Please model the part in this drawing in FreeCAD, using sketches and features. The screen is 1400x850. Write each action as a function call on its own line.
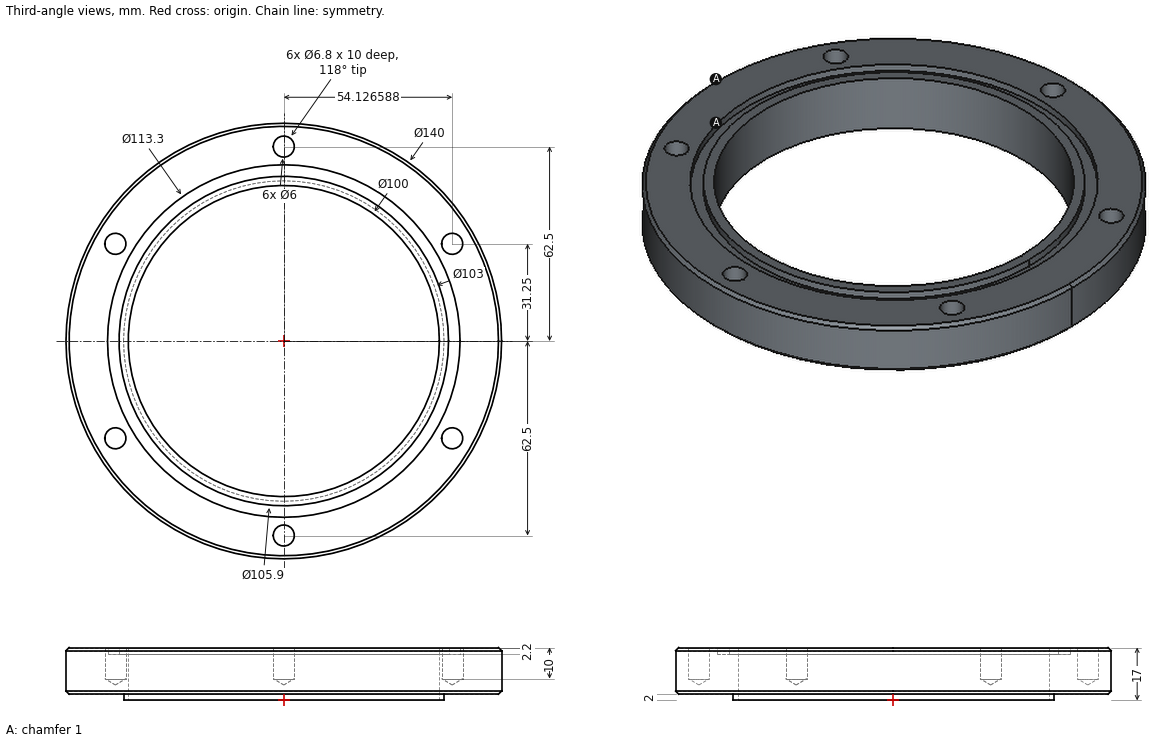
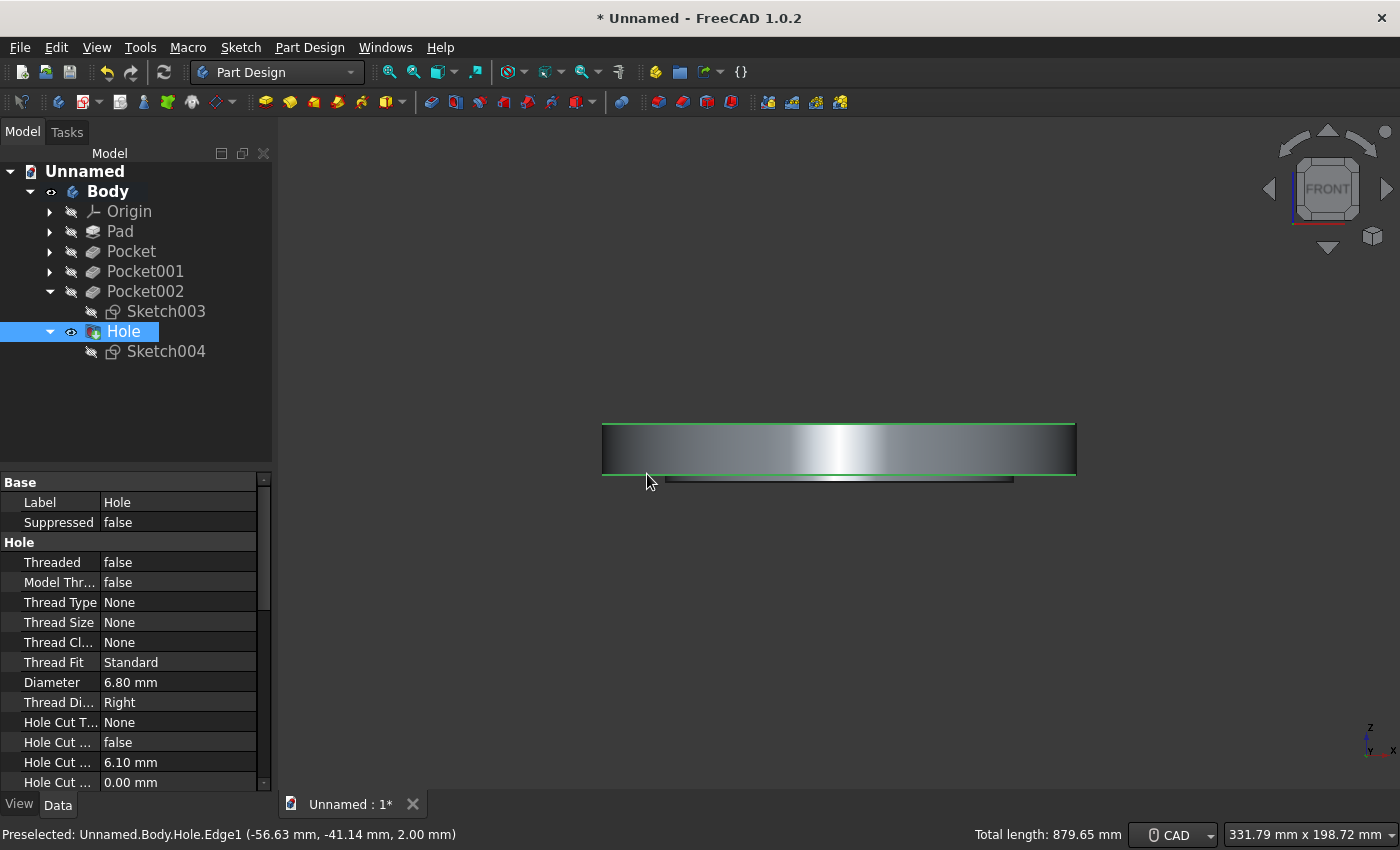
click(684, 102)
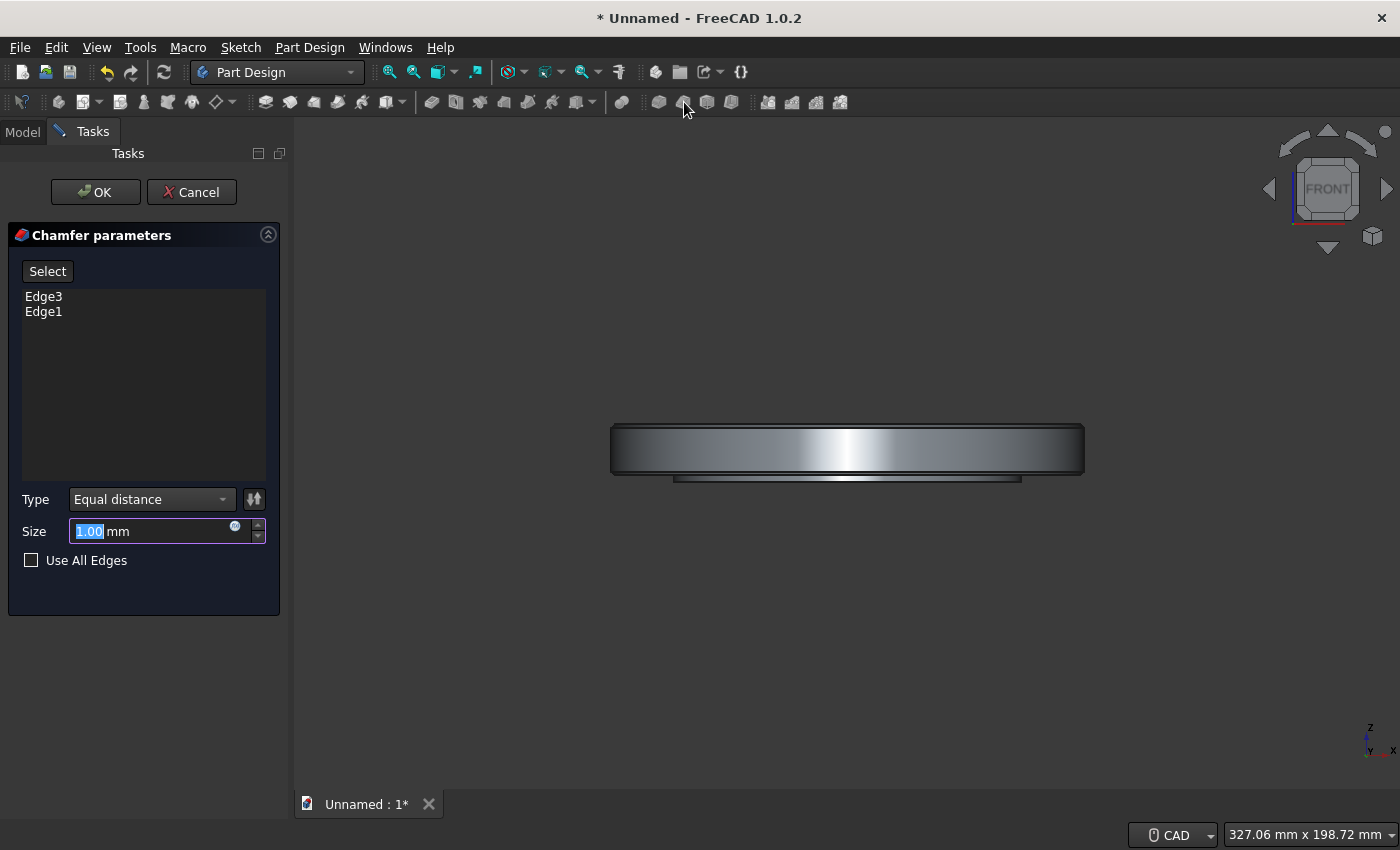
text(1)
key(Tab)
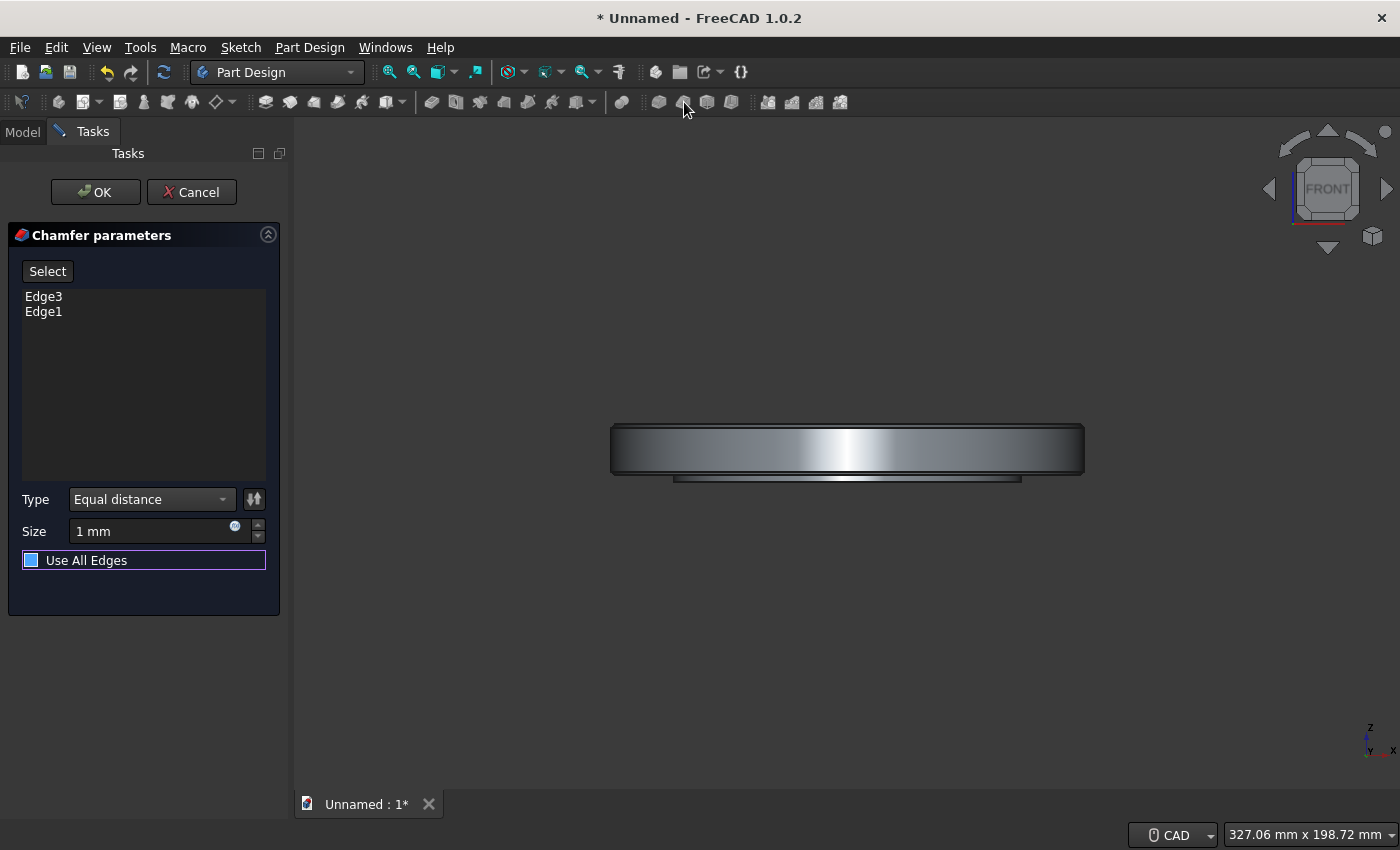
click(96, 192)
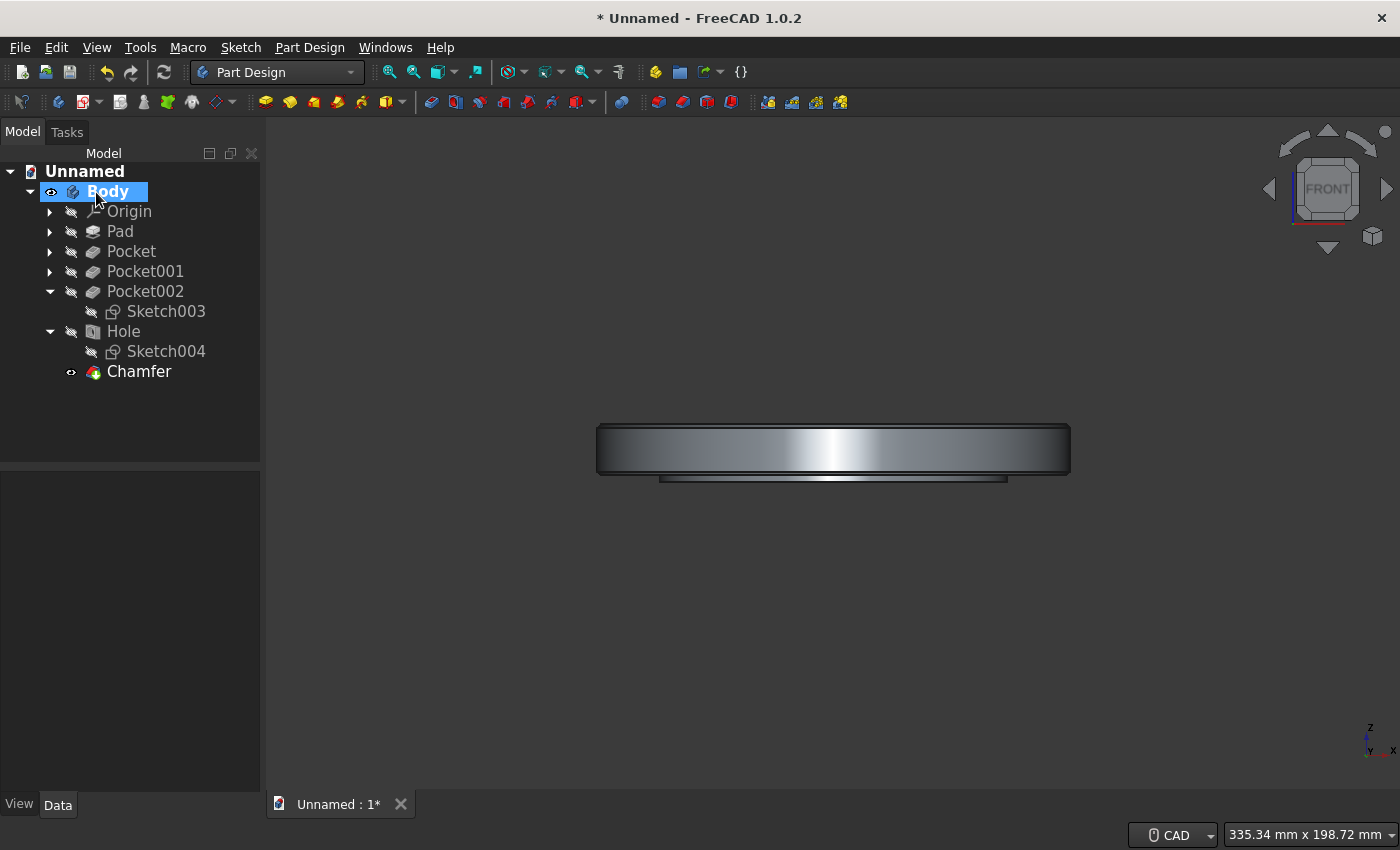
key(0)